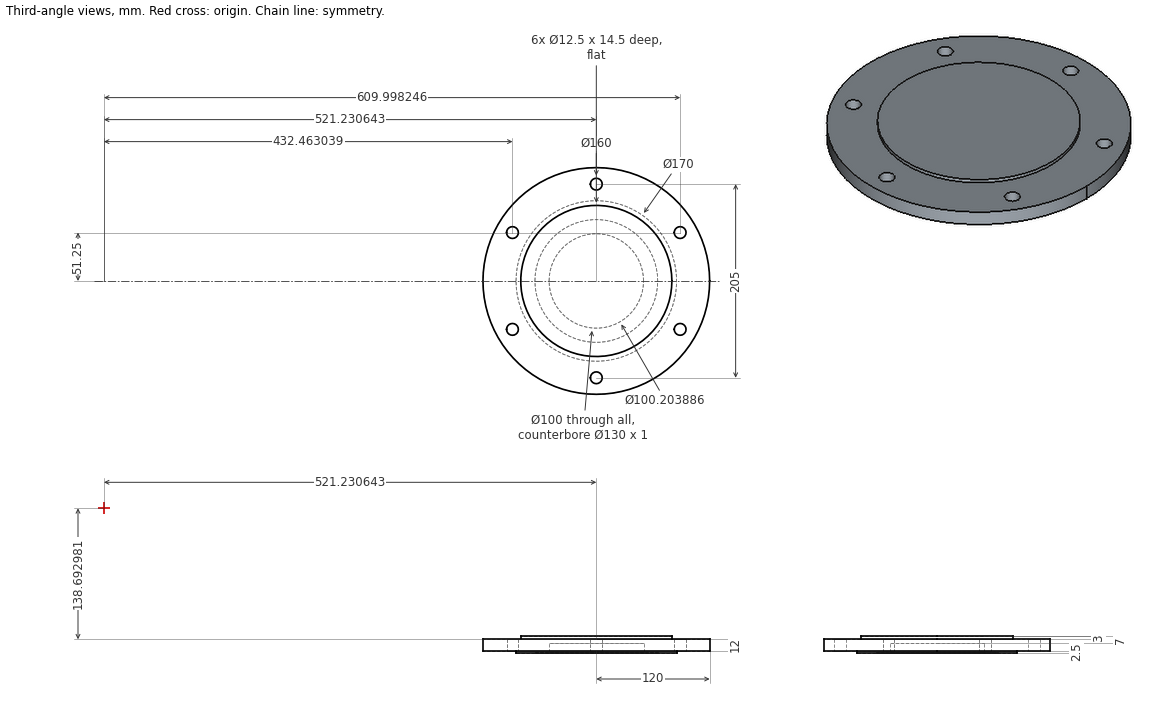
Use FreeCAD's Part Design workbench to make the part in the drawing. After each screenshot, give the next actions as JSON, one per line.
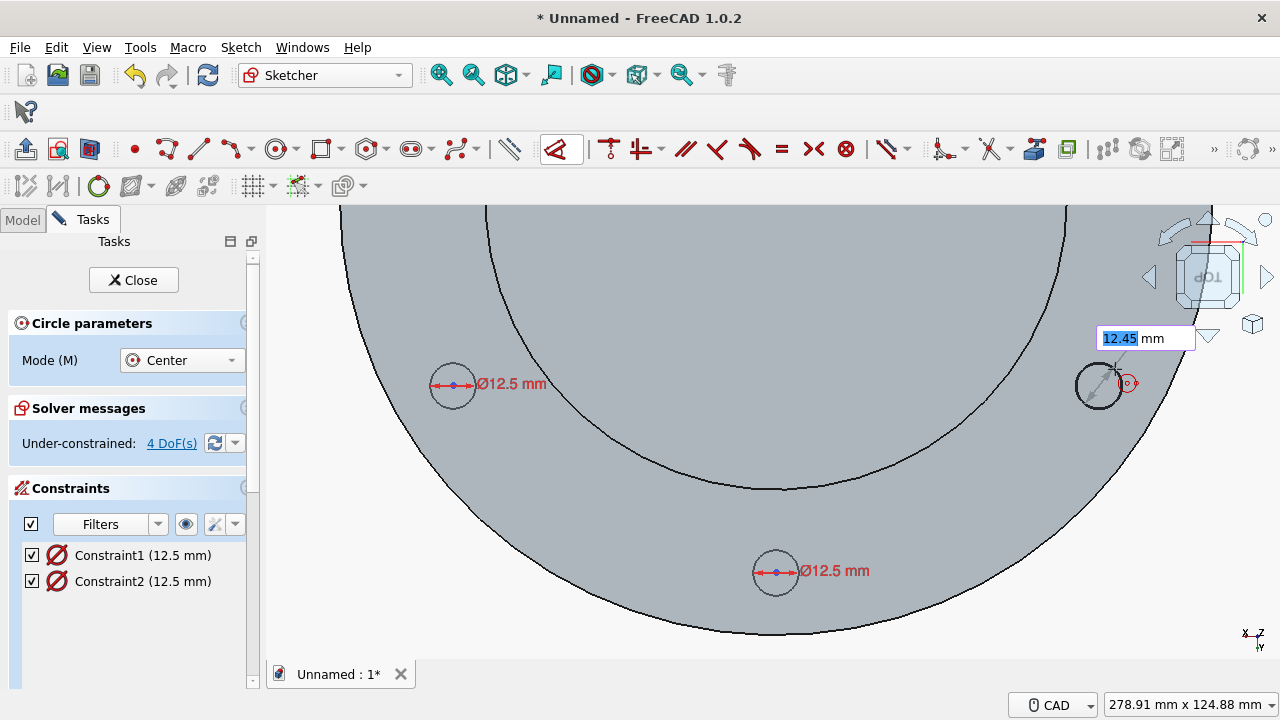
{"action": "type", "text": "12.5"}
{"action": "key", "text": "Return"}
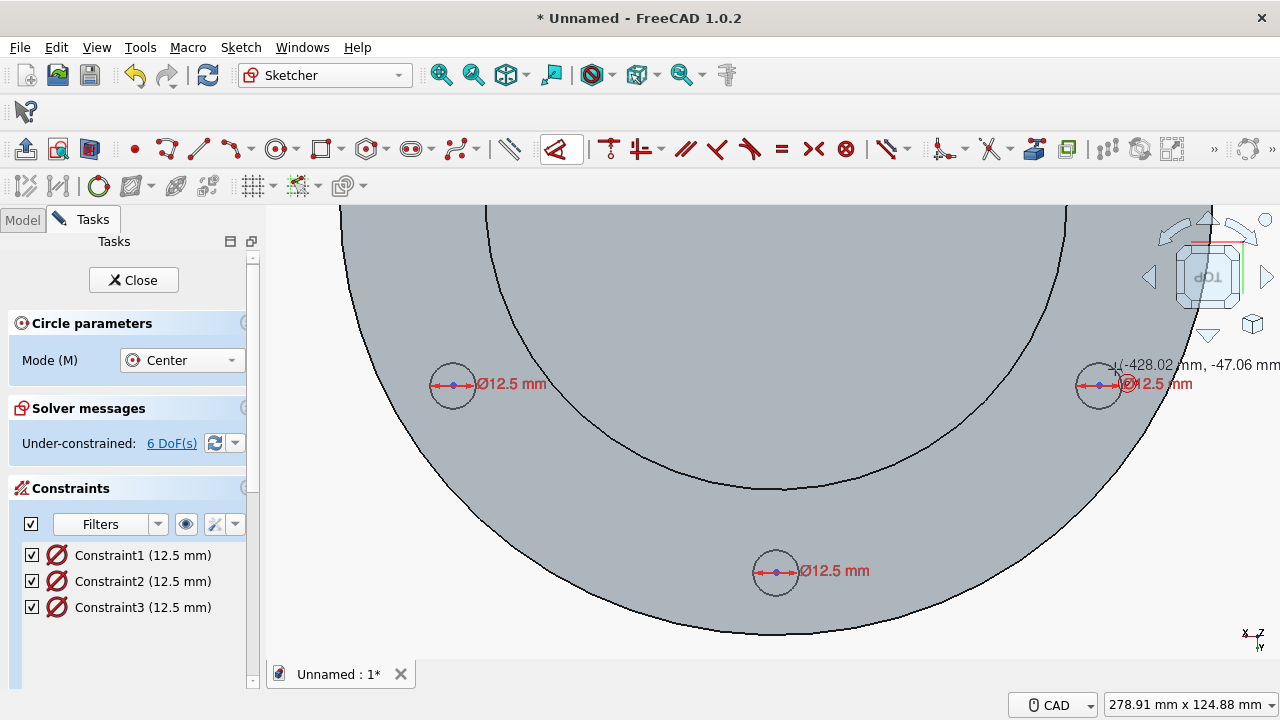
{"action": "scroll", "coordinate": [663, 568], "scroll_direction": "down", "scroll_amount": 5}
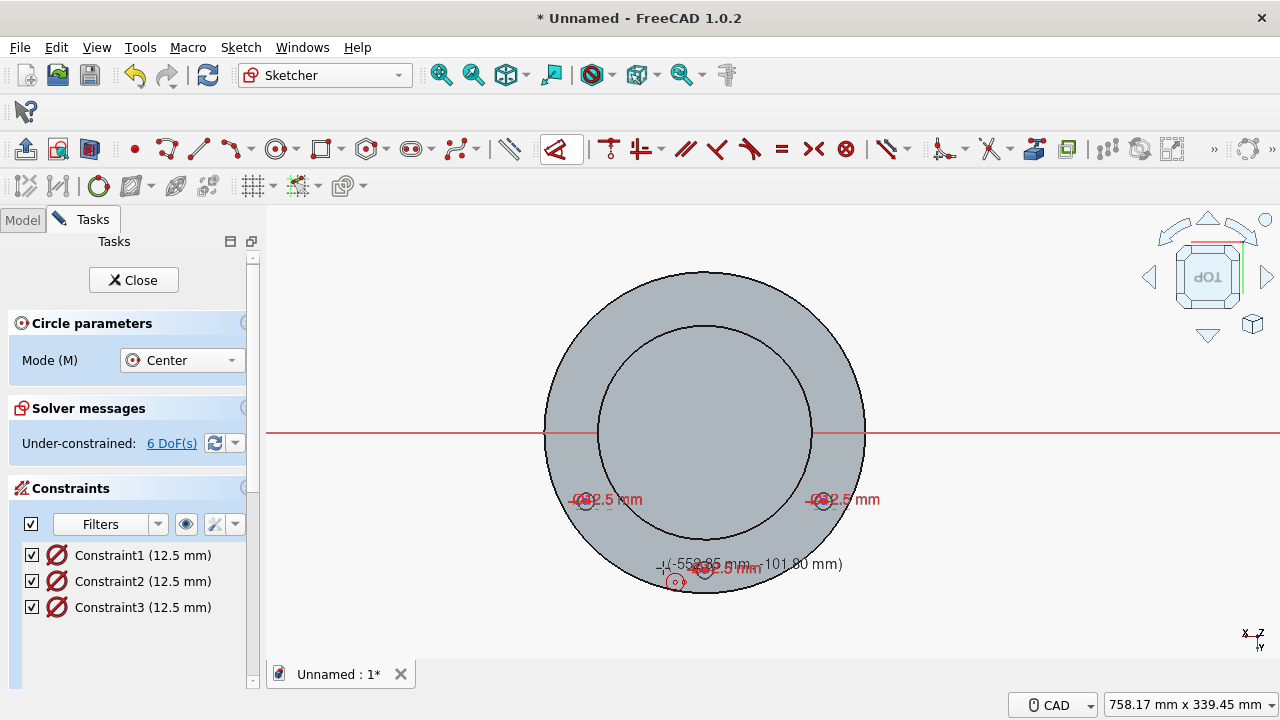
{"action": "scroll", "coordinate": [824, 364], "scroll_direction": "up", "scroll_amount": 5}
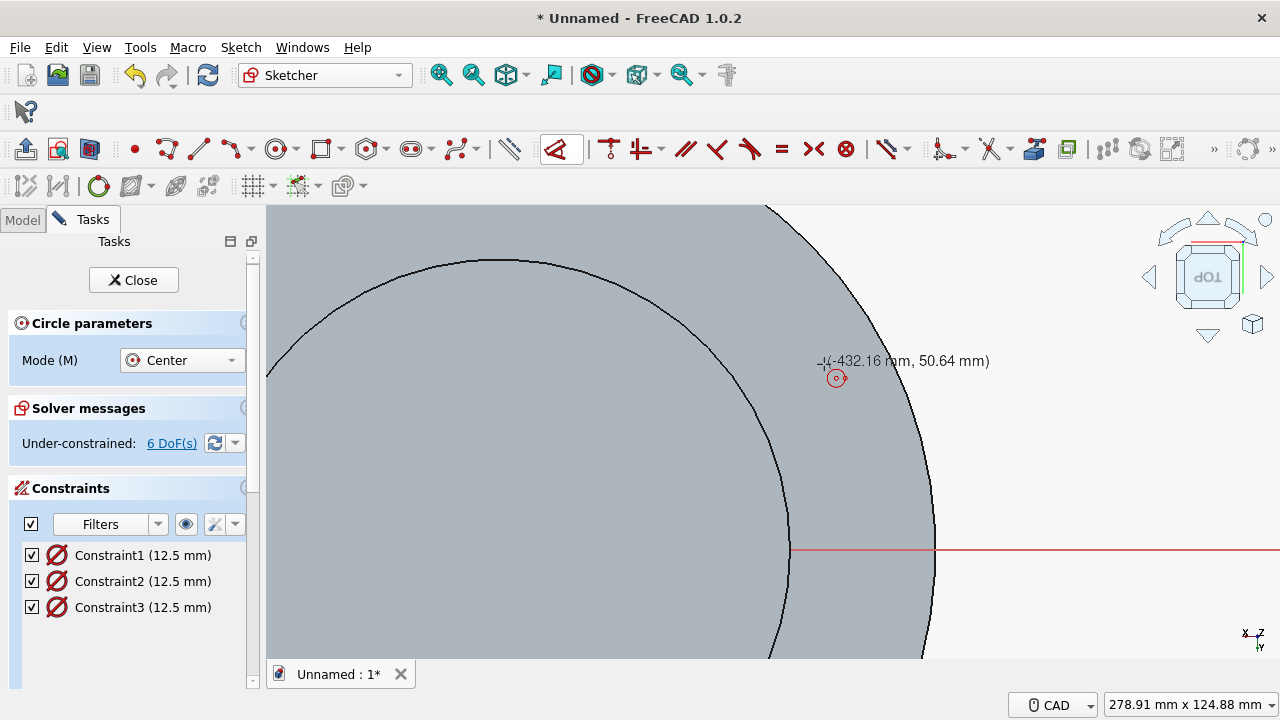
{"action": "left_click", "coordinate": [822, 364]}
{"action": "mouse_move", "coordinate": [838, 348]}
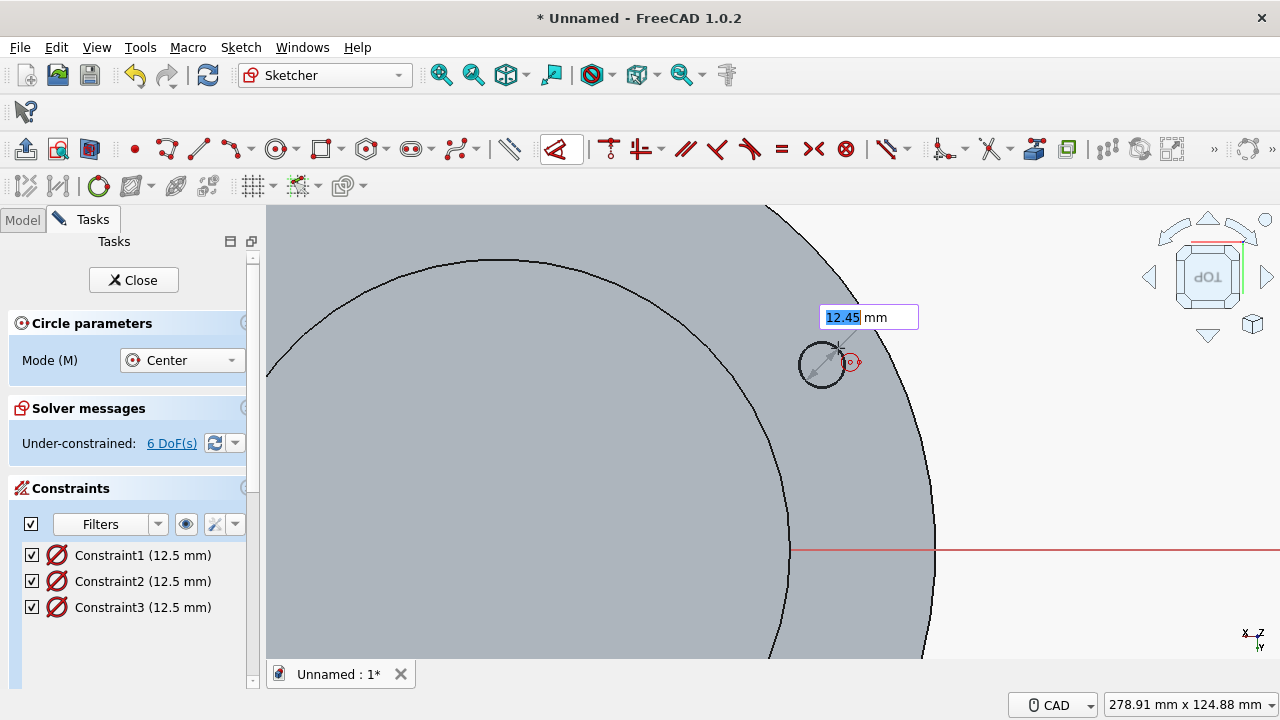
{"action": "type", "text": "12.5"}
{"action": "key", "text": "Return"}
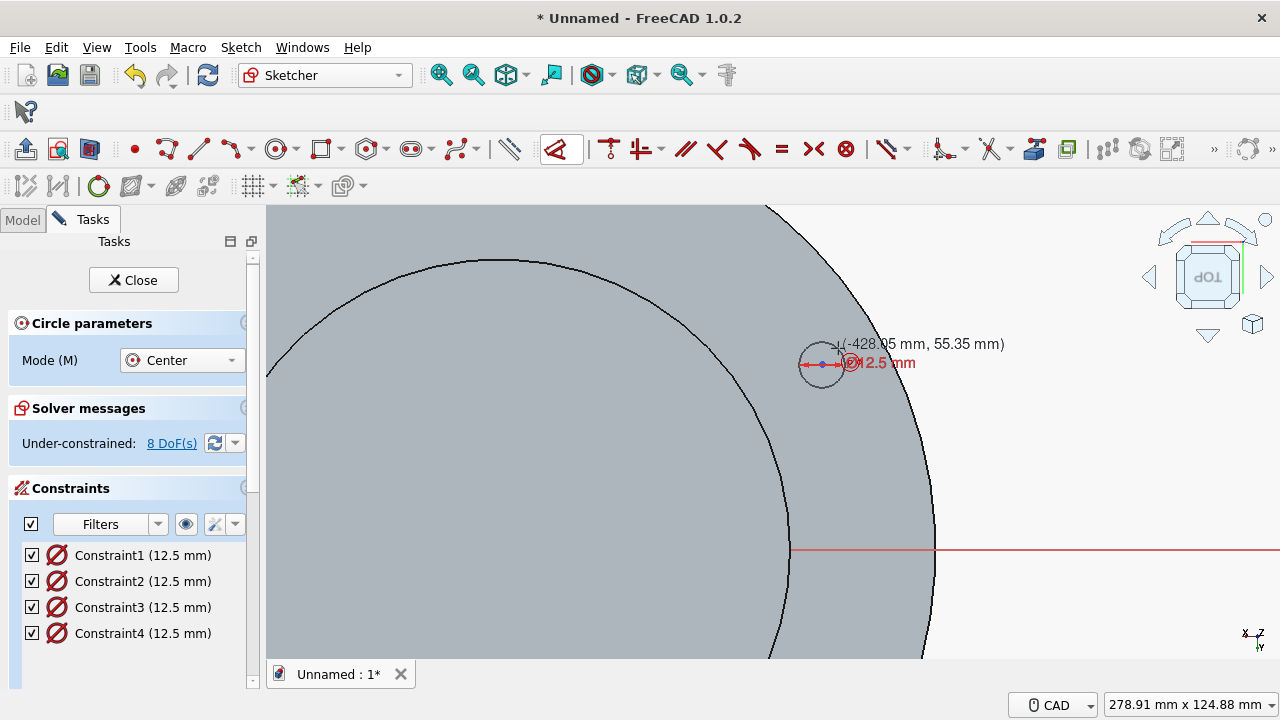
{"action": "scroll", "coordinate": [824, 363], "scroll_direction": "down", "scroll_amount": 5}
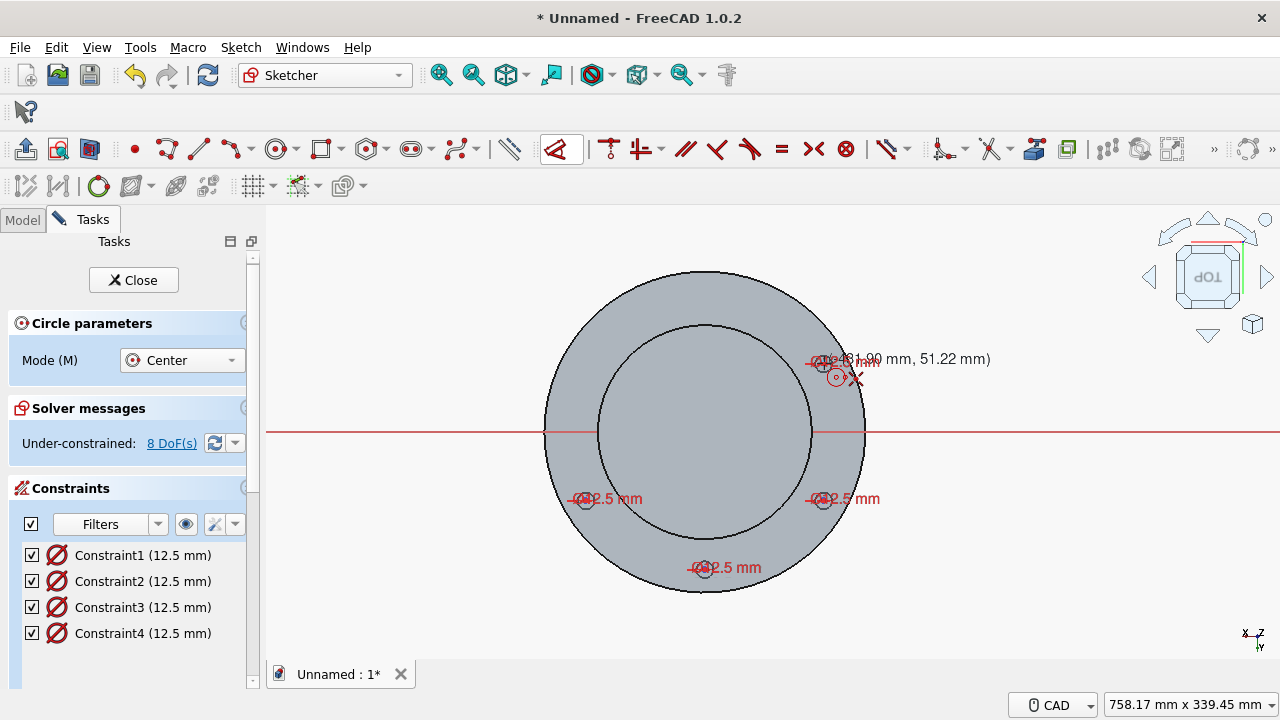
{"action": "scroll", "coordinate": [705, 295], "scroll_direction": "up", "scroll_amount": 5}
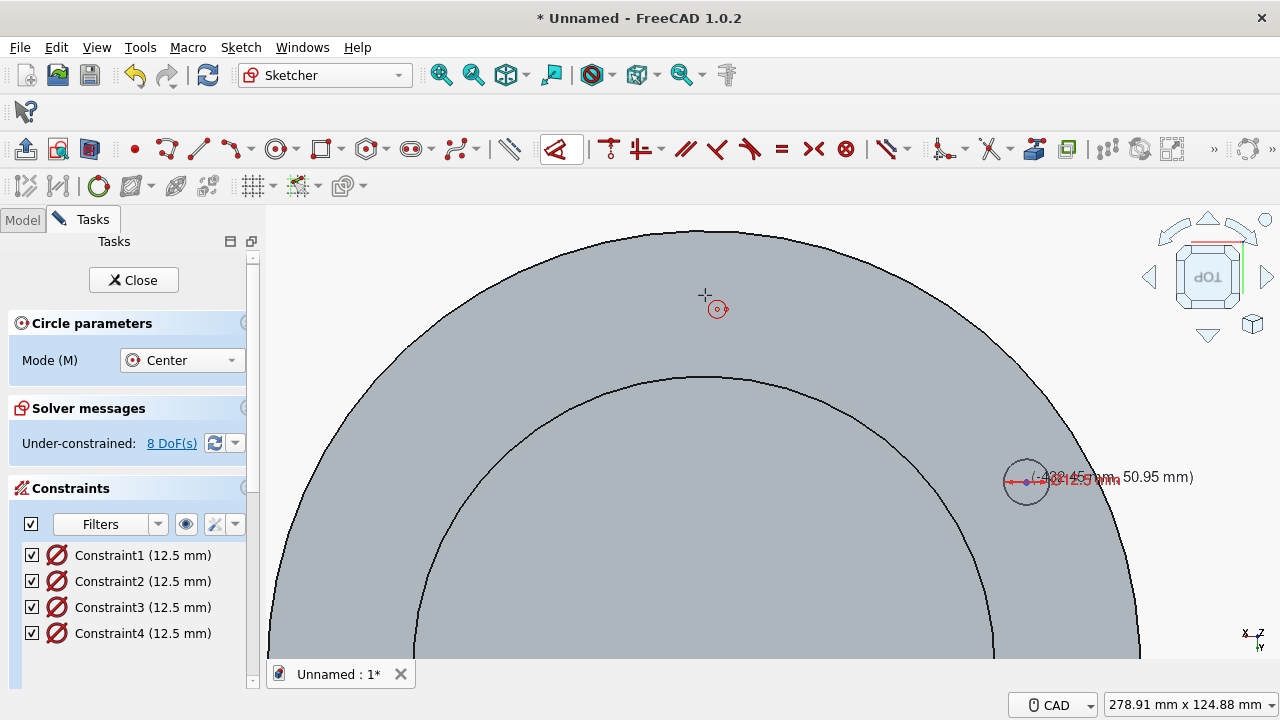
{"action": "left_click", "coordinate": [704, 295]}
{"action": "mouse_move", "coordinate": [720, 279]}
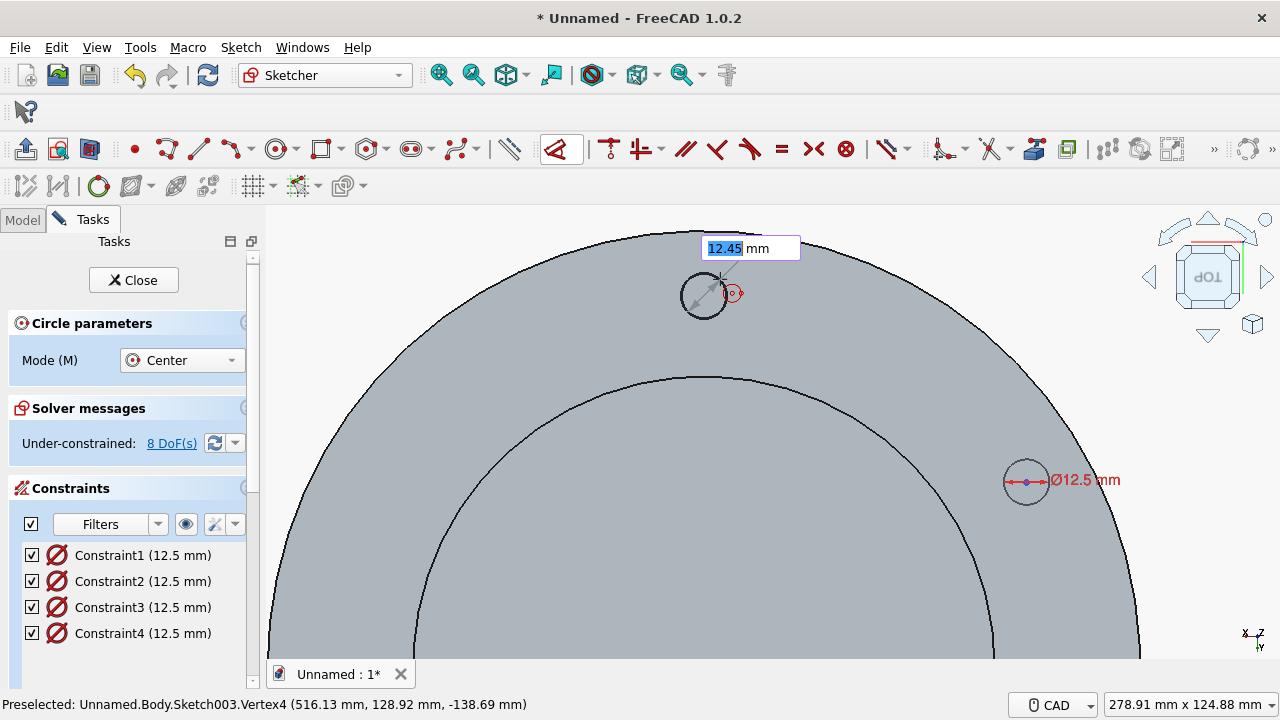
{"action": "type", "text": "12.5"}
{"action": "key", "text": "Return"}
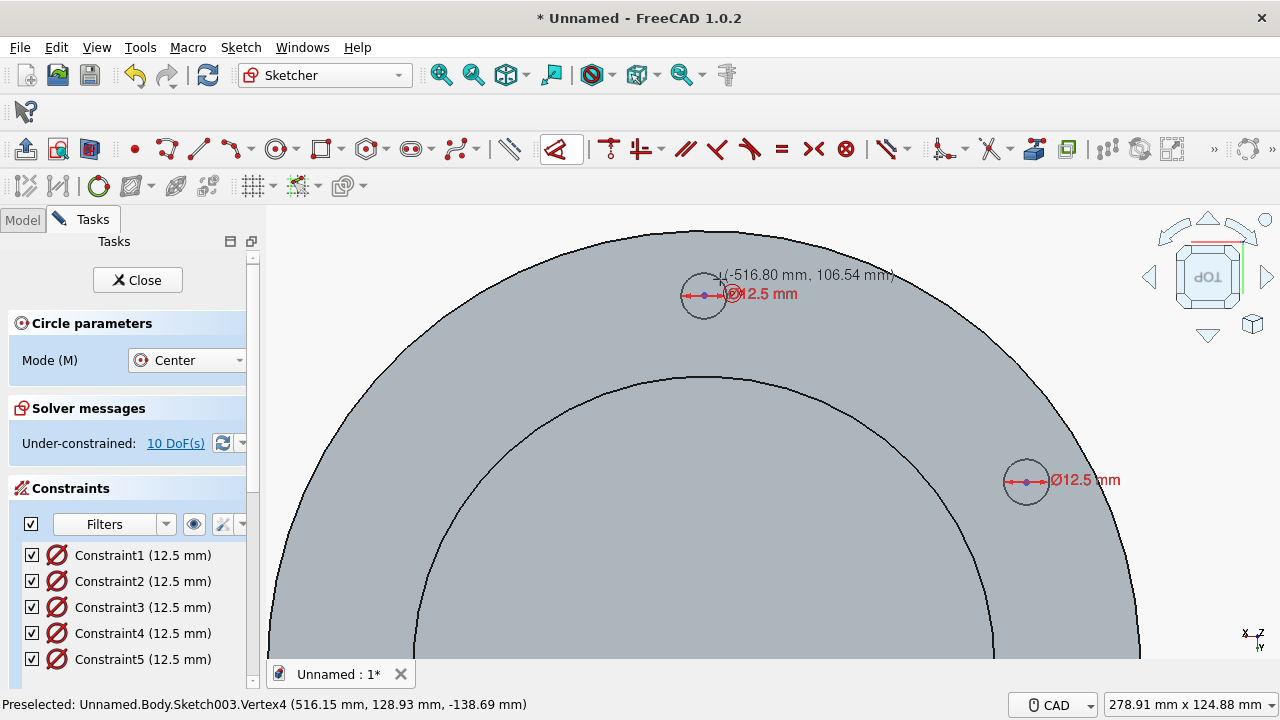
{"action": "left_click", "coordinate": [381, 481]}
{"action": "mouse_move", "coordinate": [397, 465]}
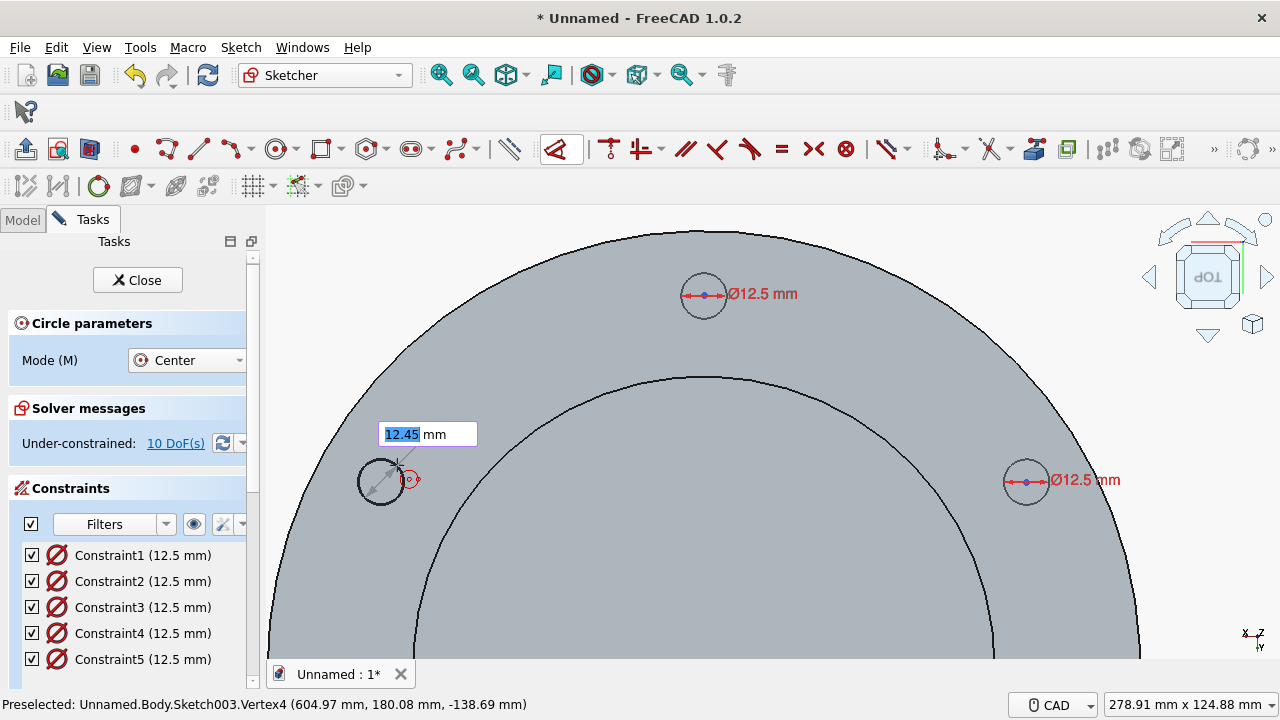
{"action": "type", "text": "12.5"}
{"action": "key", "text": "Return"}
{"action": "key", "text": "Escape"}